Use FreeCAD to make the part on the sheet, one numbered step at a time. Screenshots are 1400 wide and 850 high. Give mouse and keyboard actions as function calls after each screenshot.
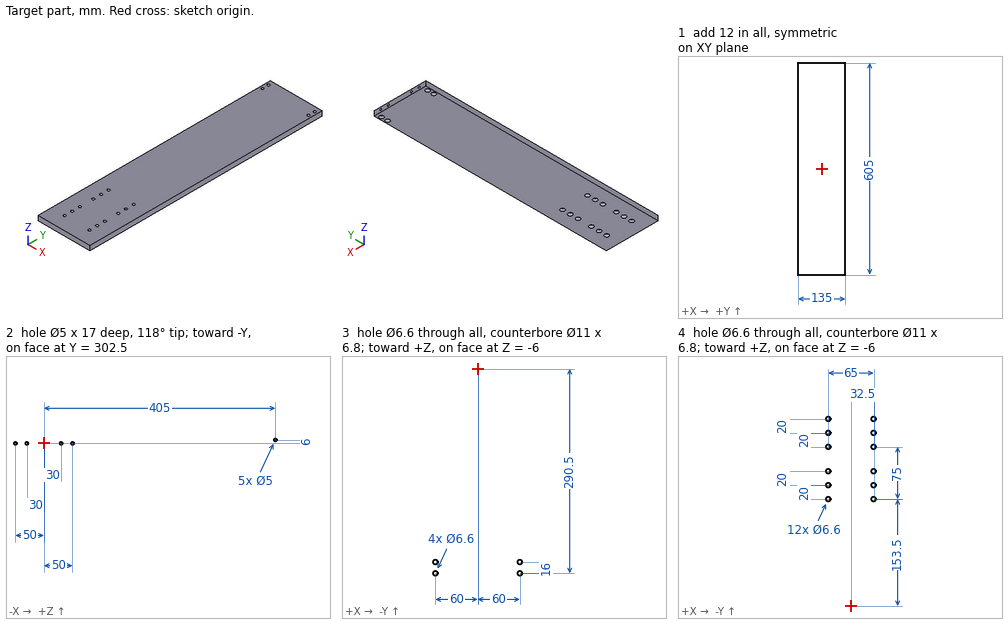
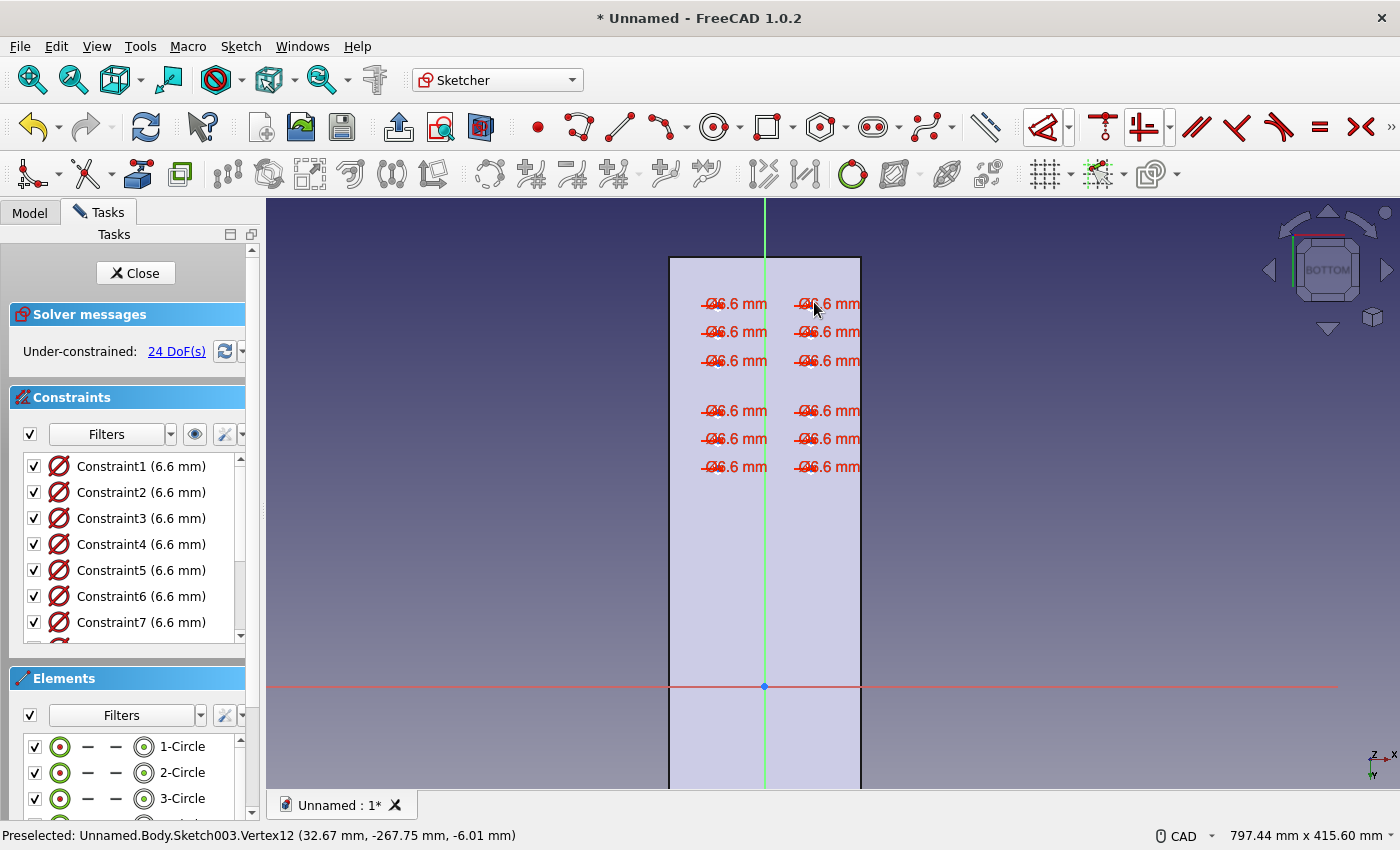
click(811, 469)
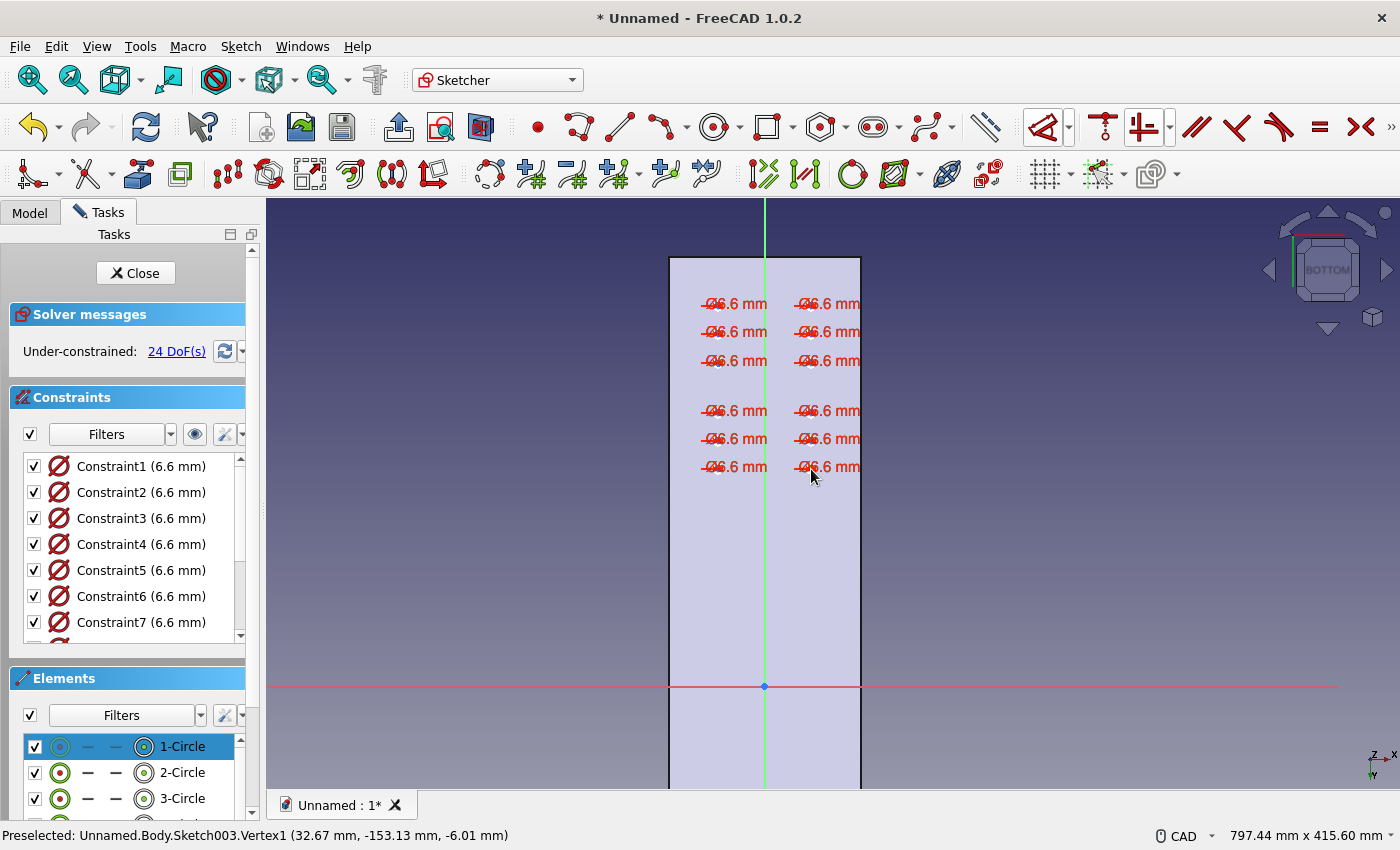
click(811, 363)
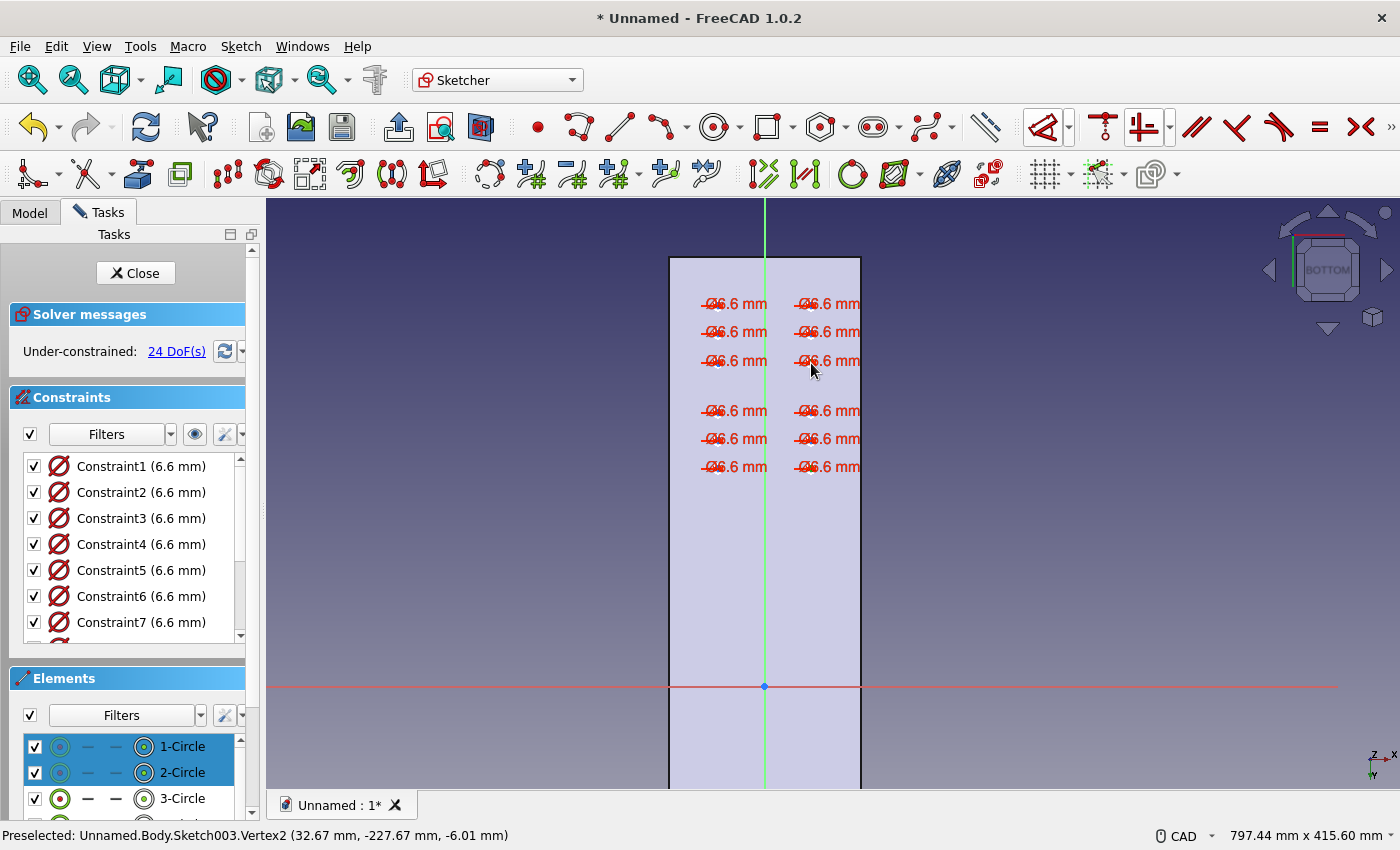
key(v)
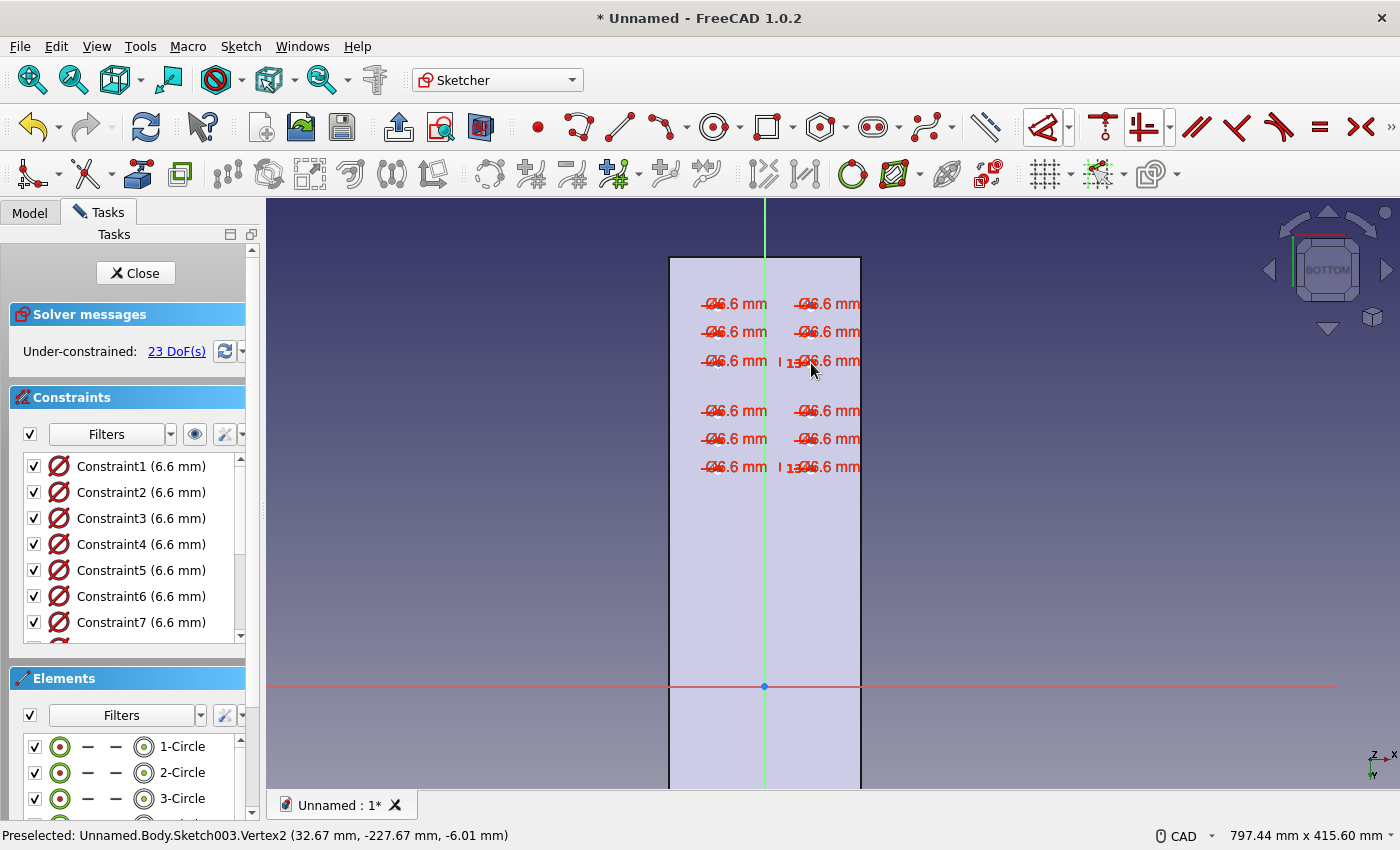
click(811, 363)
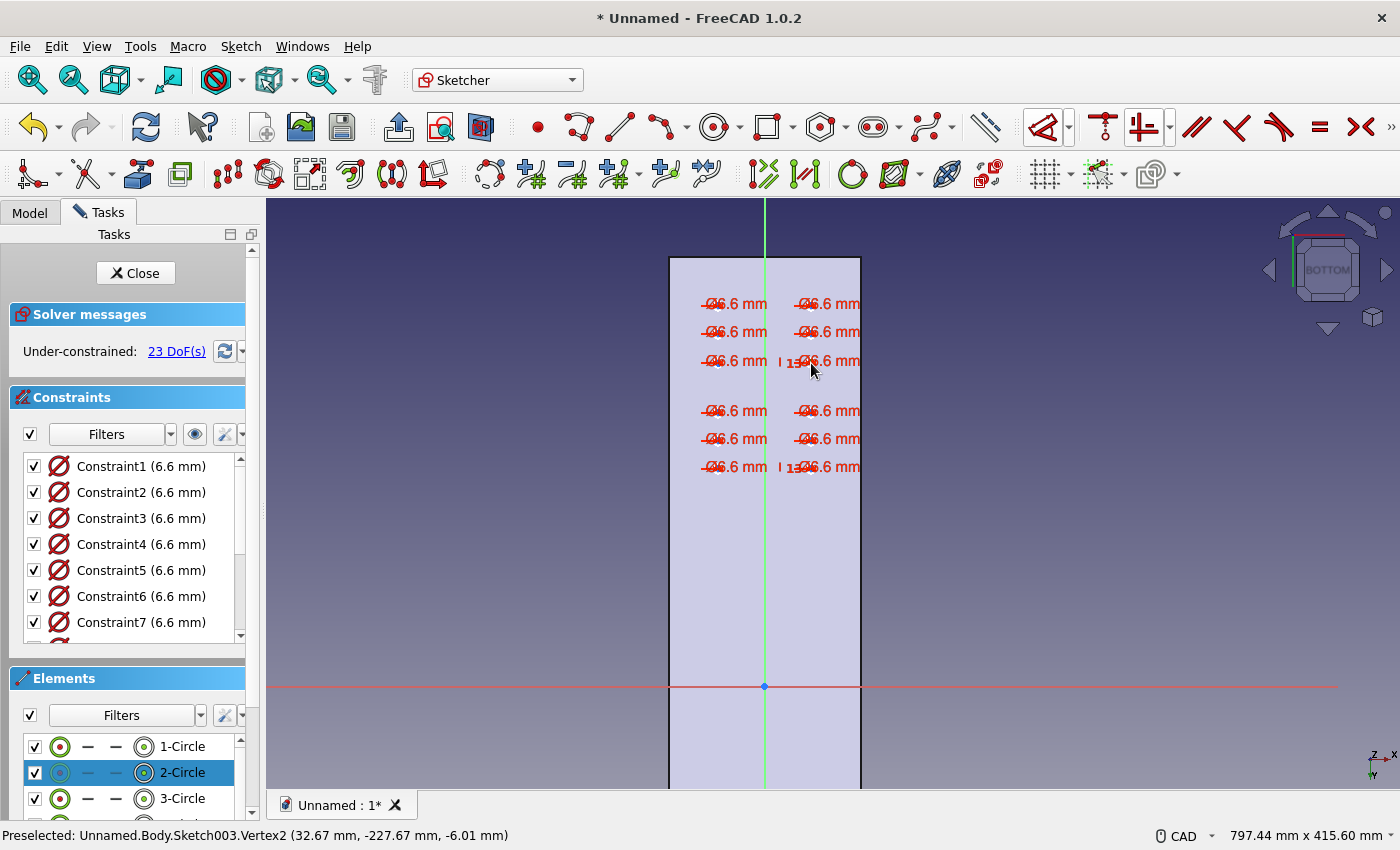
click(718, 363)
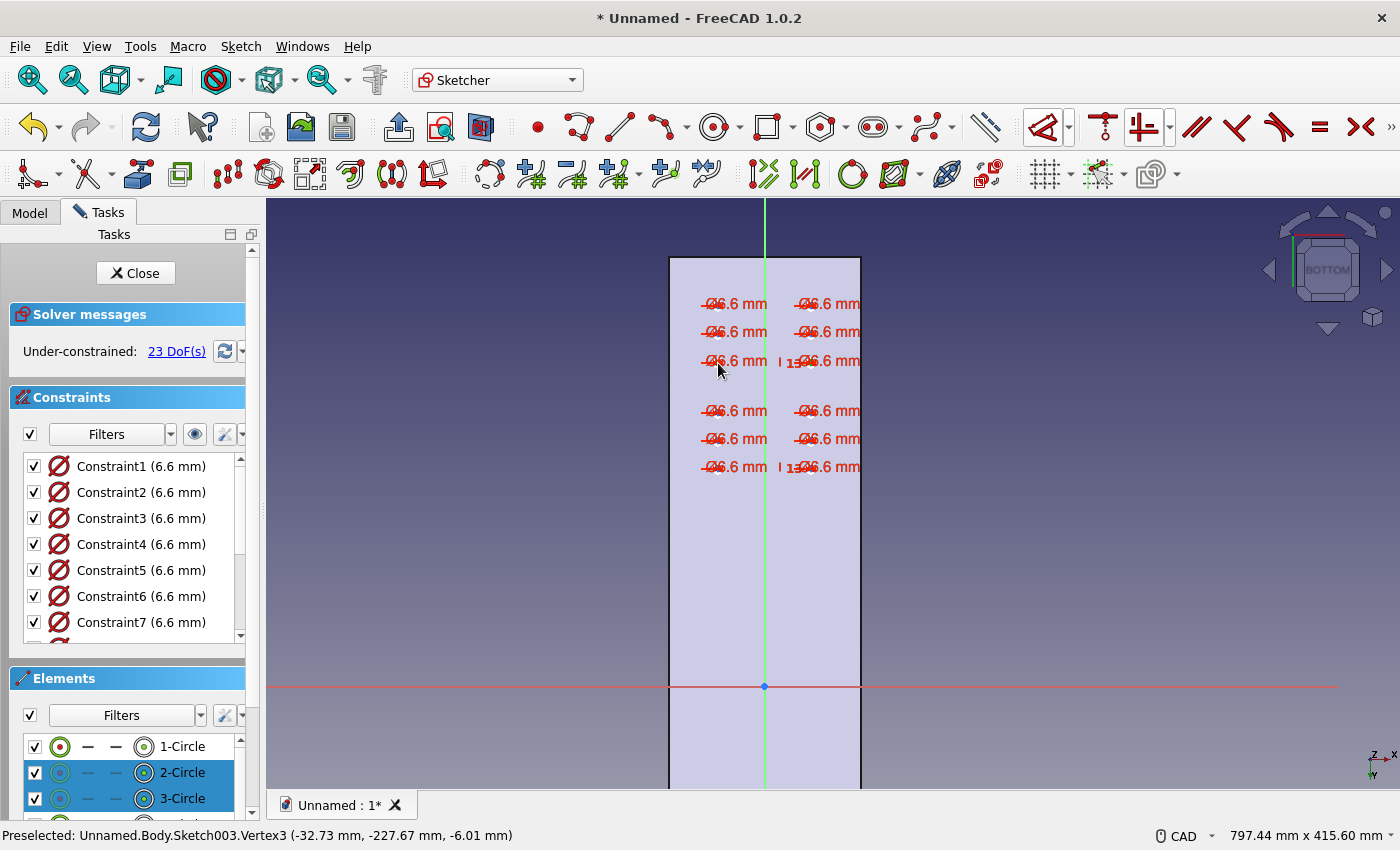
click(1170, 128)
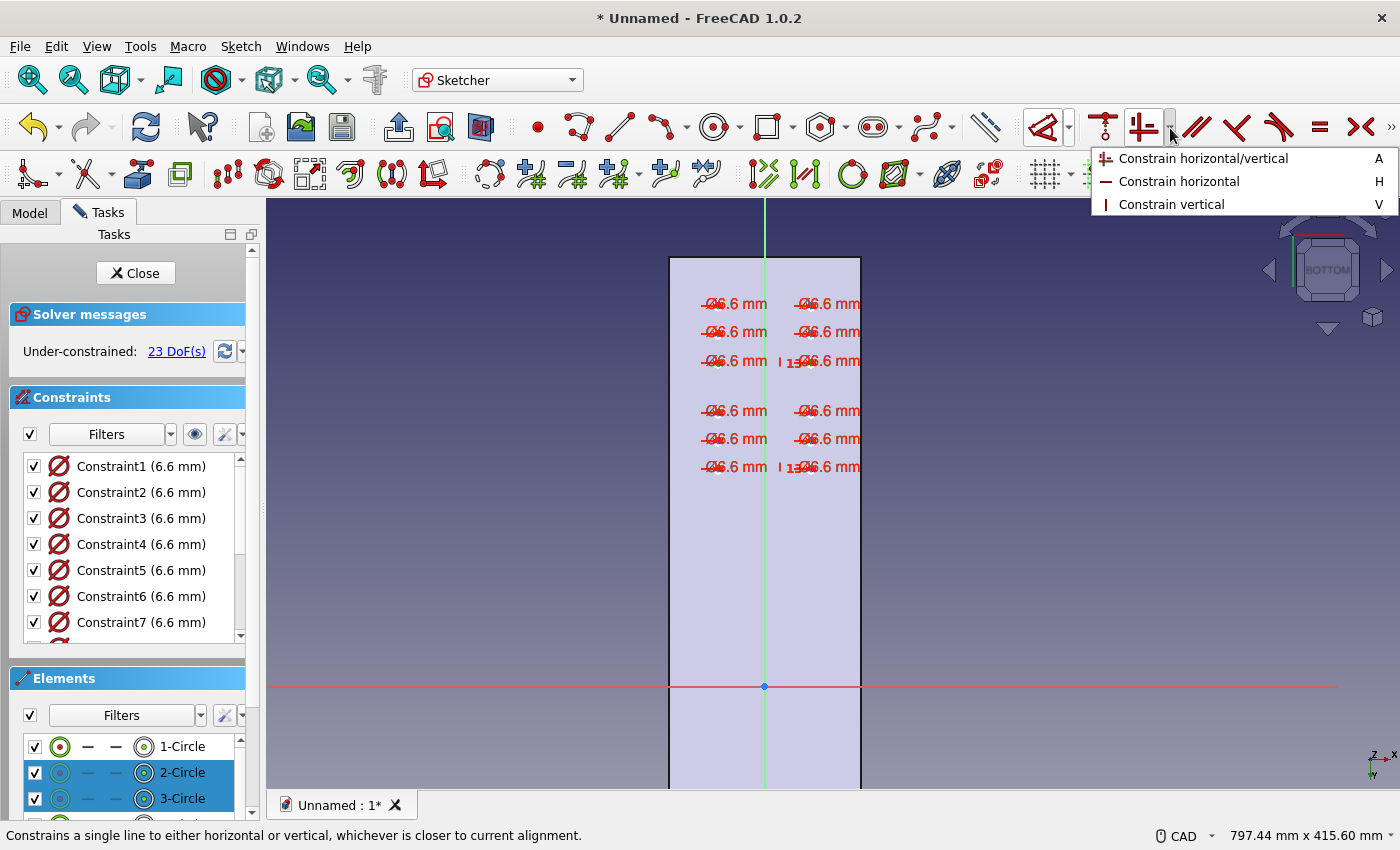
click(1245, 182)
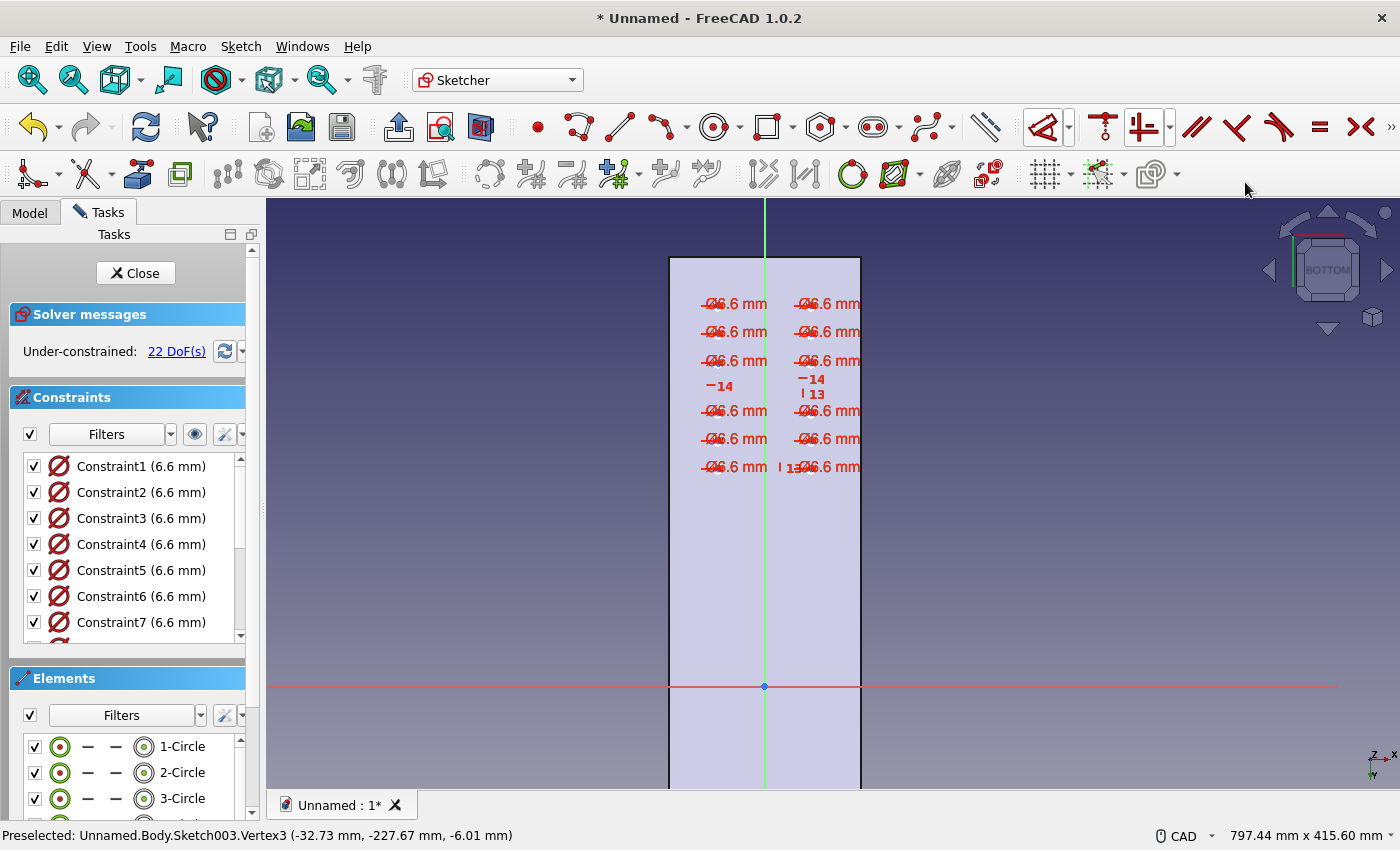
click(718, 363)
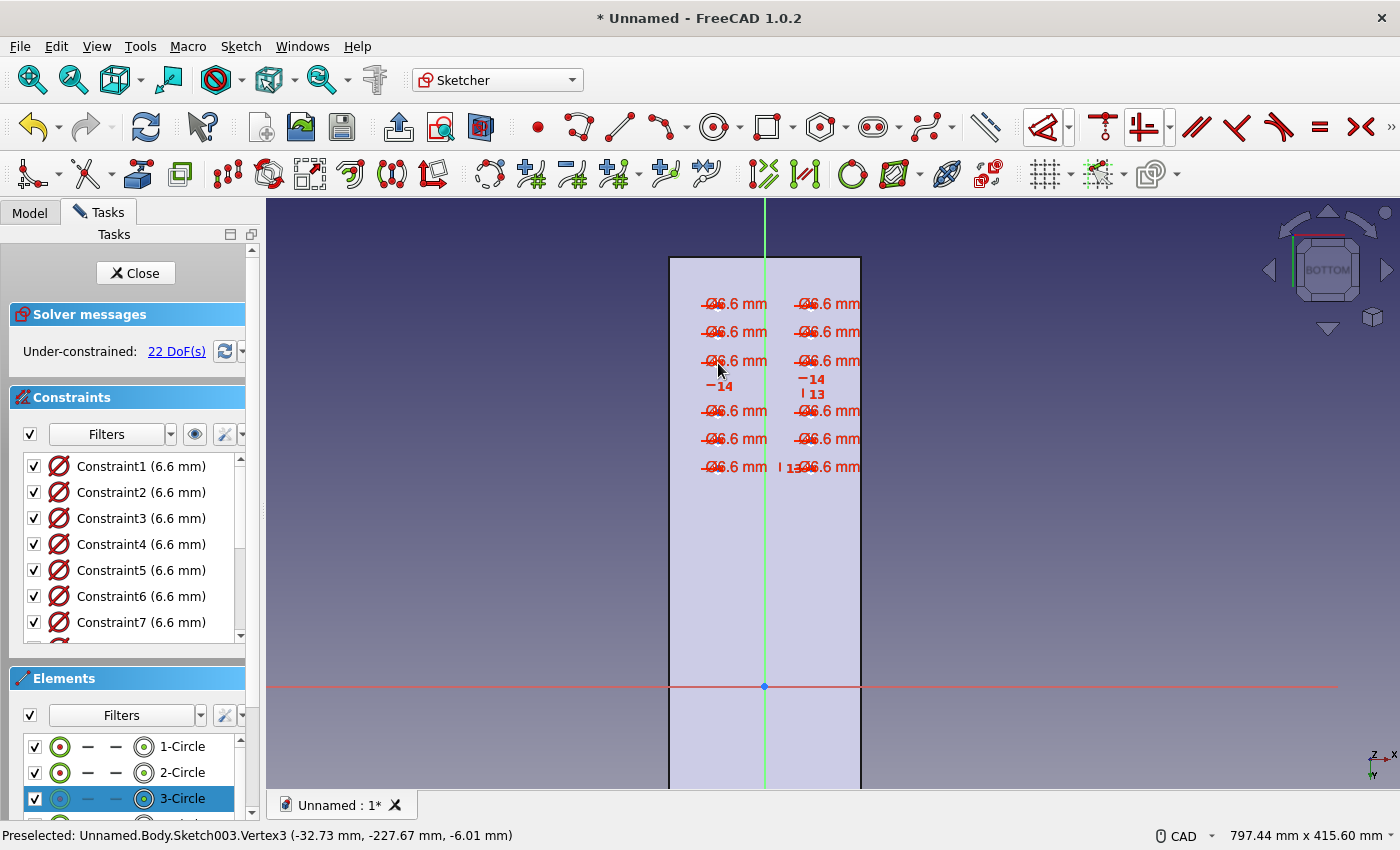
click(718, 469)